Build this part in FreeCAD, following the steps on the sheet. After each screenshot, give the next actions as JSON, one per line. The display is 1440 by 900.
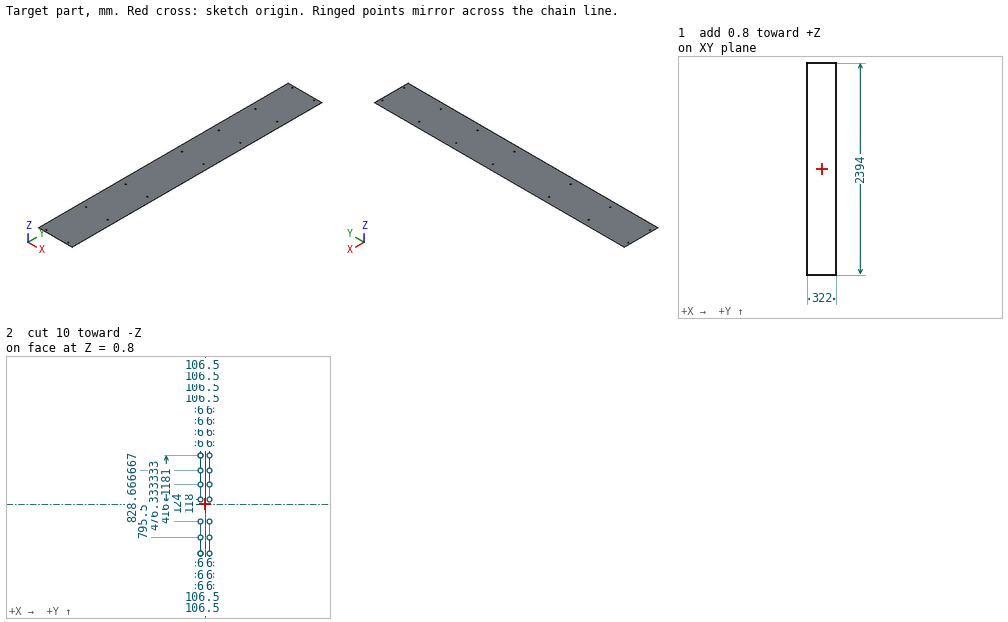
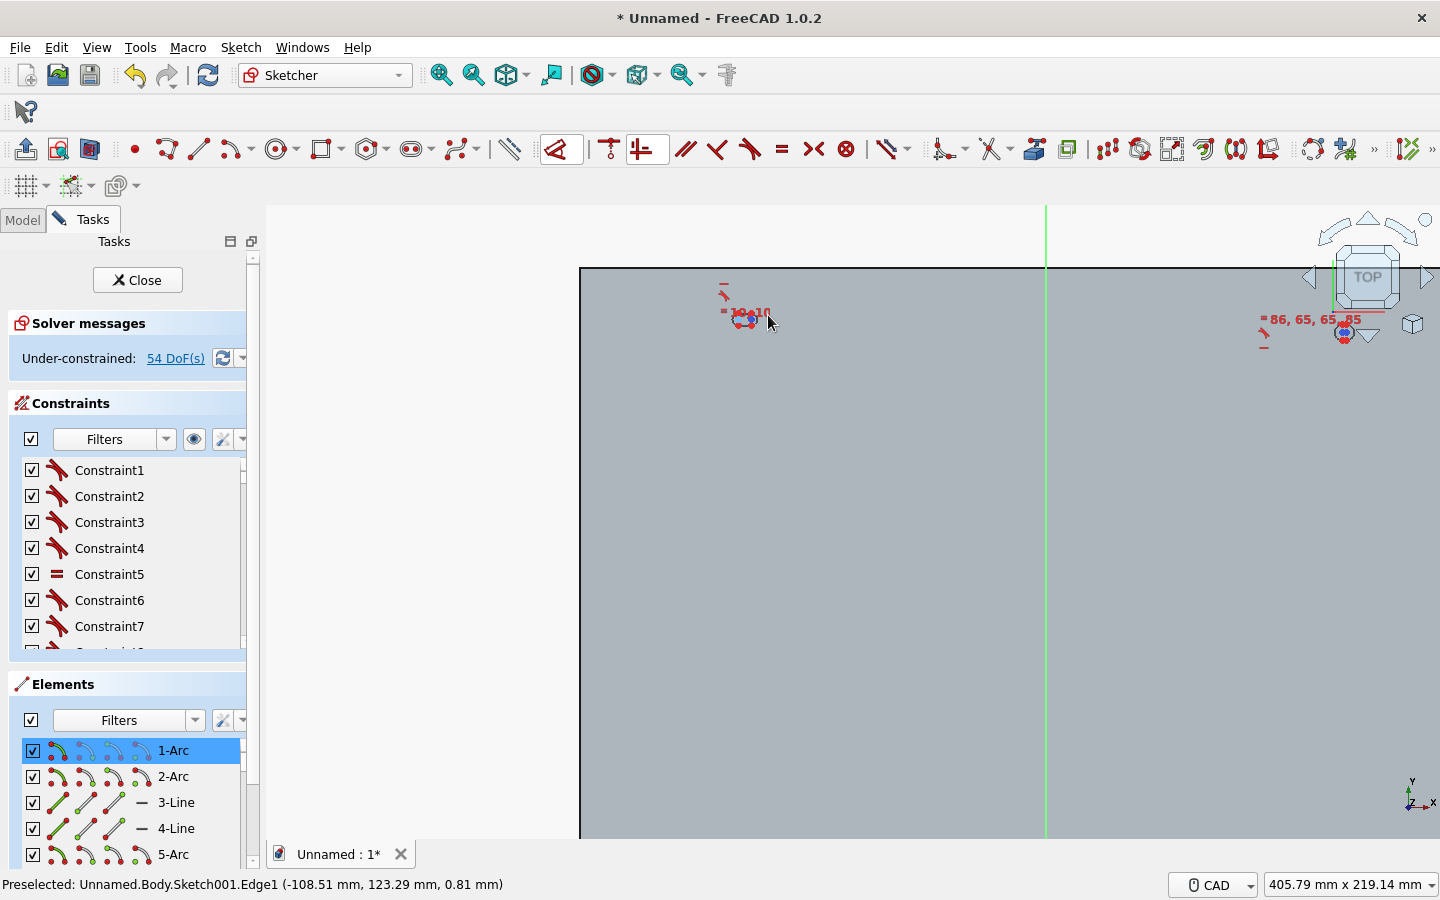
{"action": "left_click", "coordinate": [757, 320]}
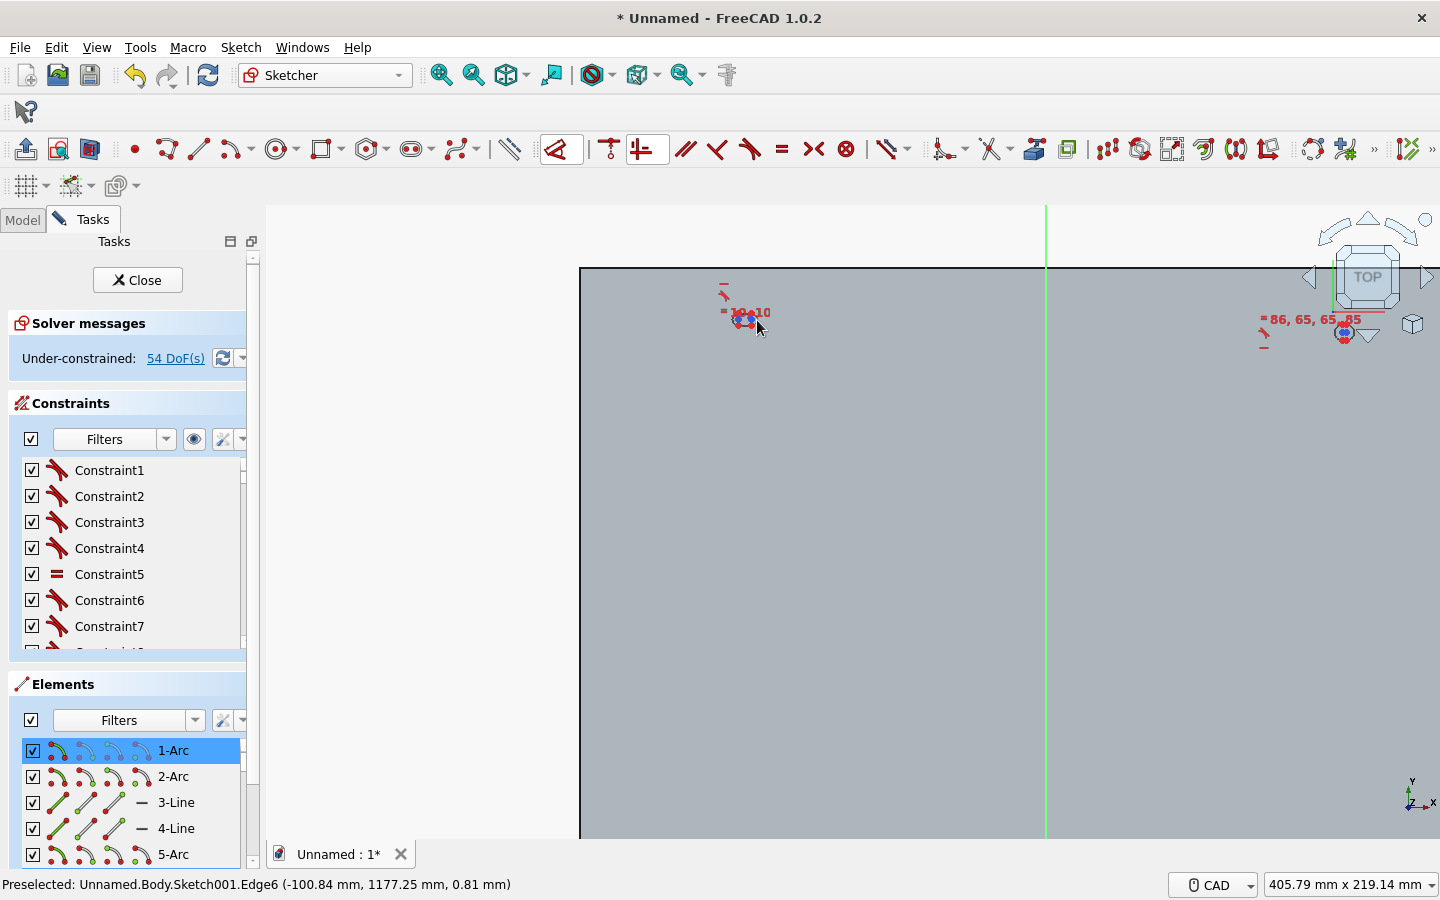
{"action": "scroll", "coordinate": [768, 314], "scroll_direction": "down", "scroll_amount": 14}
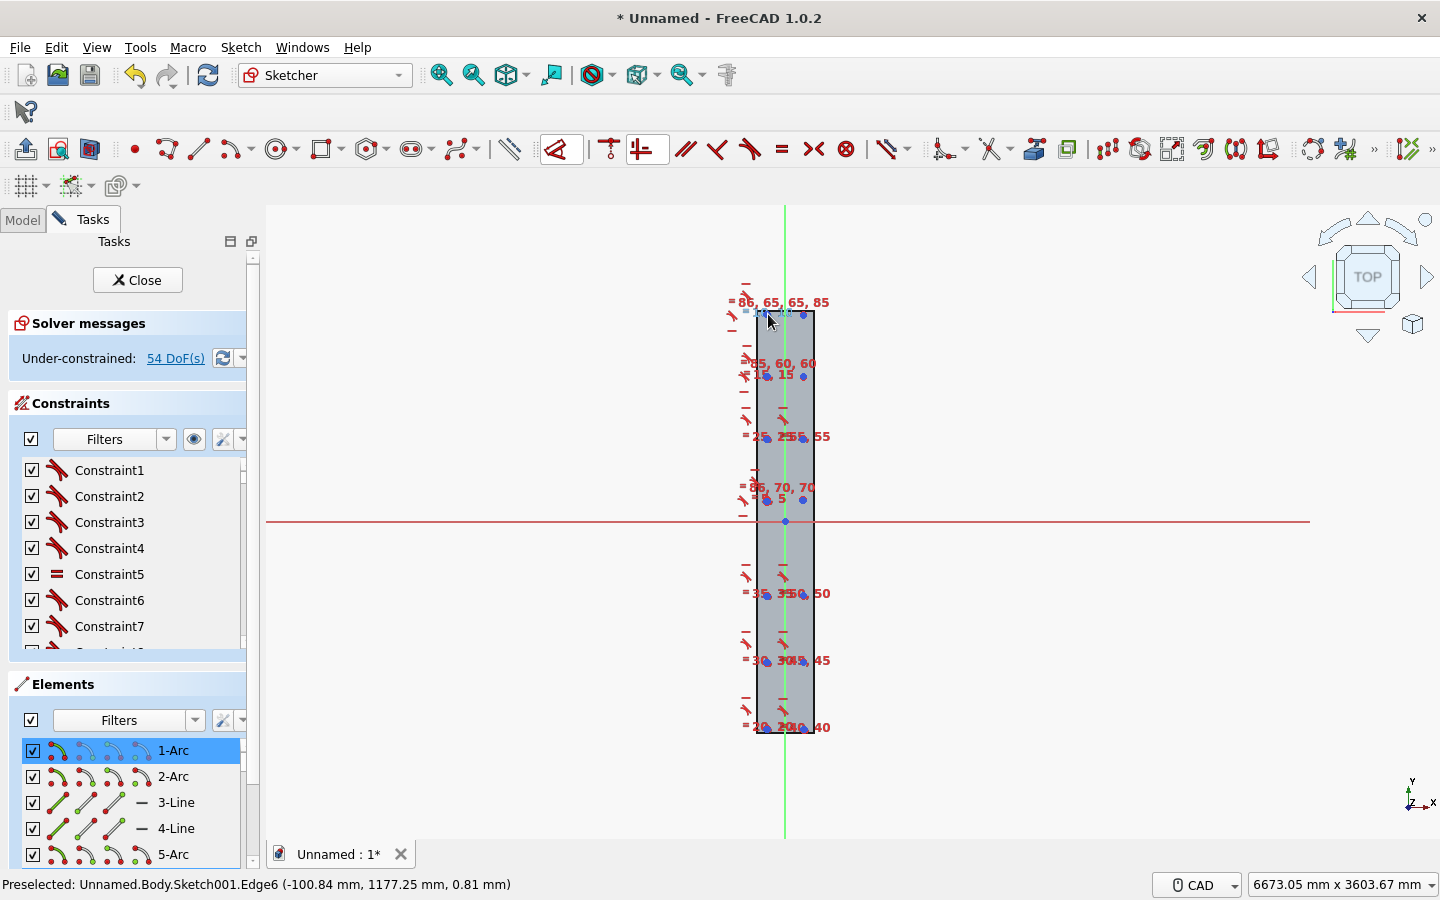
{"action": "scroll", "coordinate": [768, 377], "scroll_direction": "up", "scroll_amount": 14}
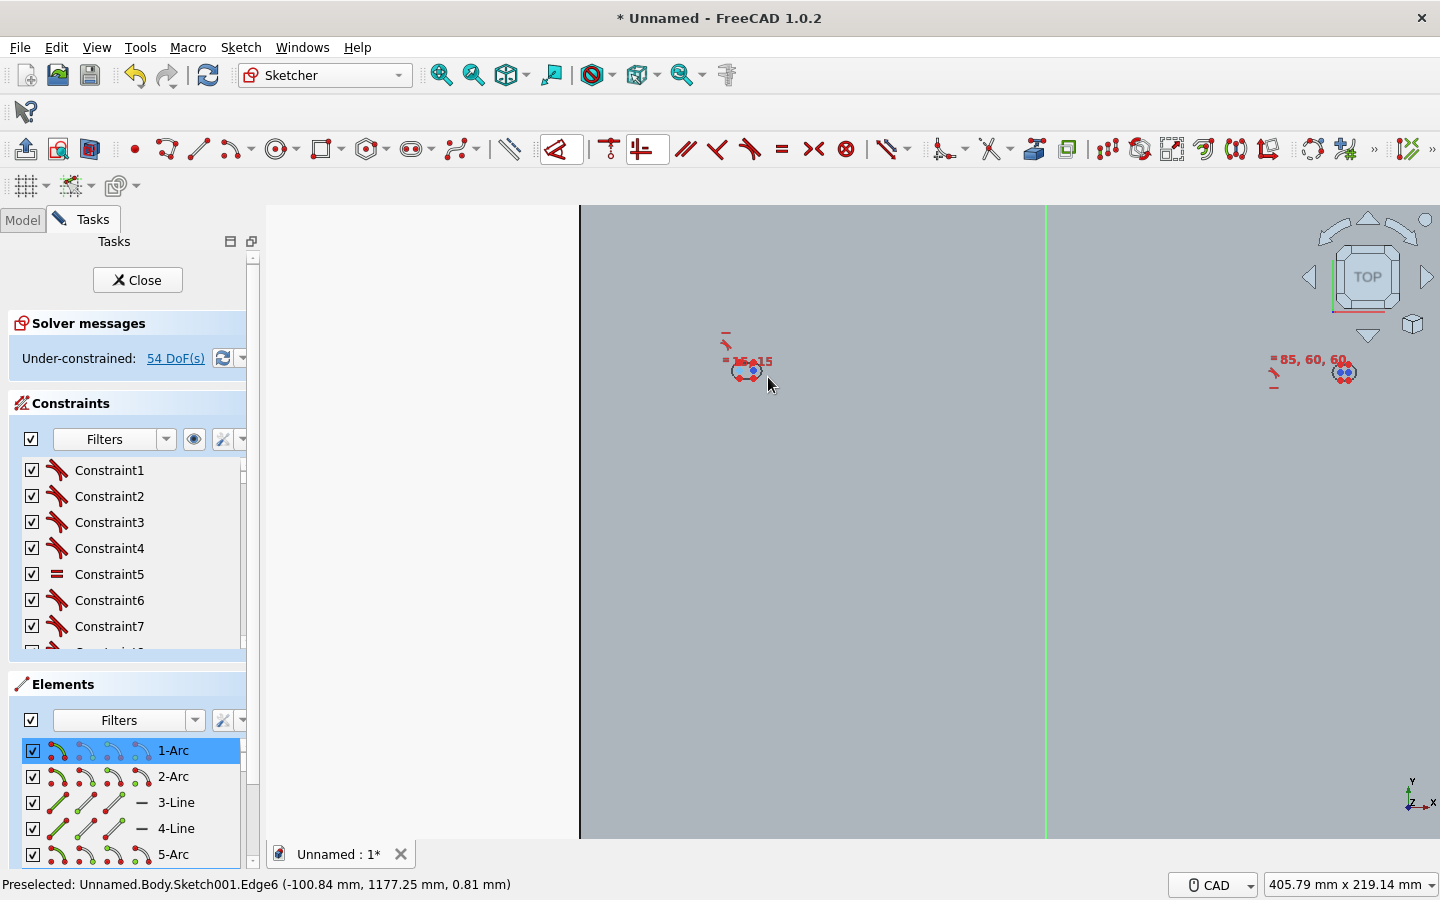
{"action": "left_click", "coordinate": [762, 371]}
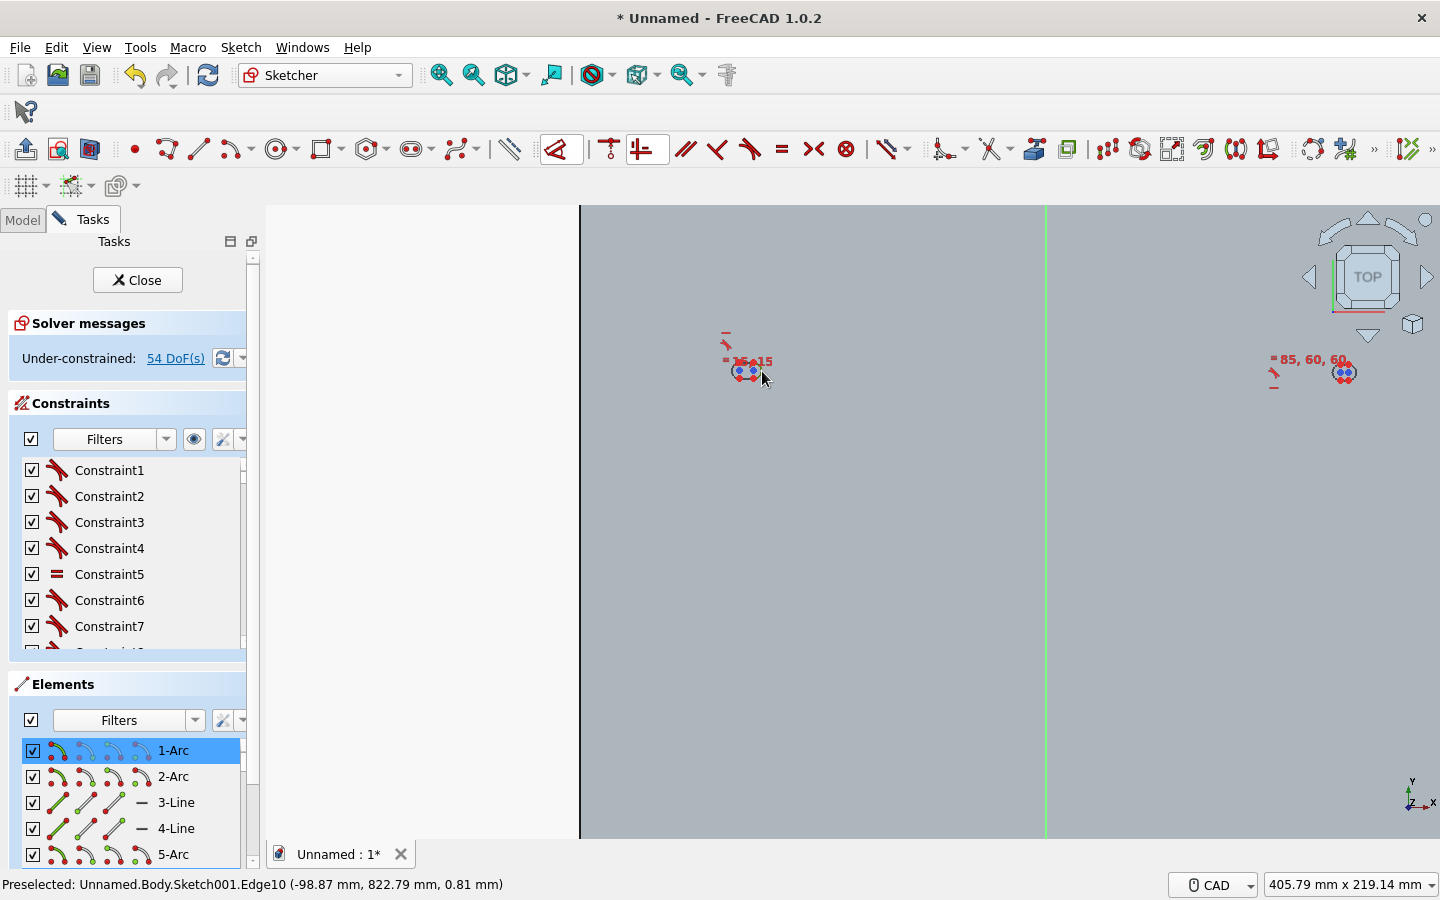
{"action": "scroll", "coordinate": [768, 377], "scroll_direction": "down", "scroll_amount": 14}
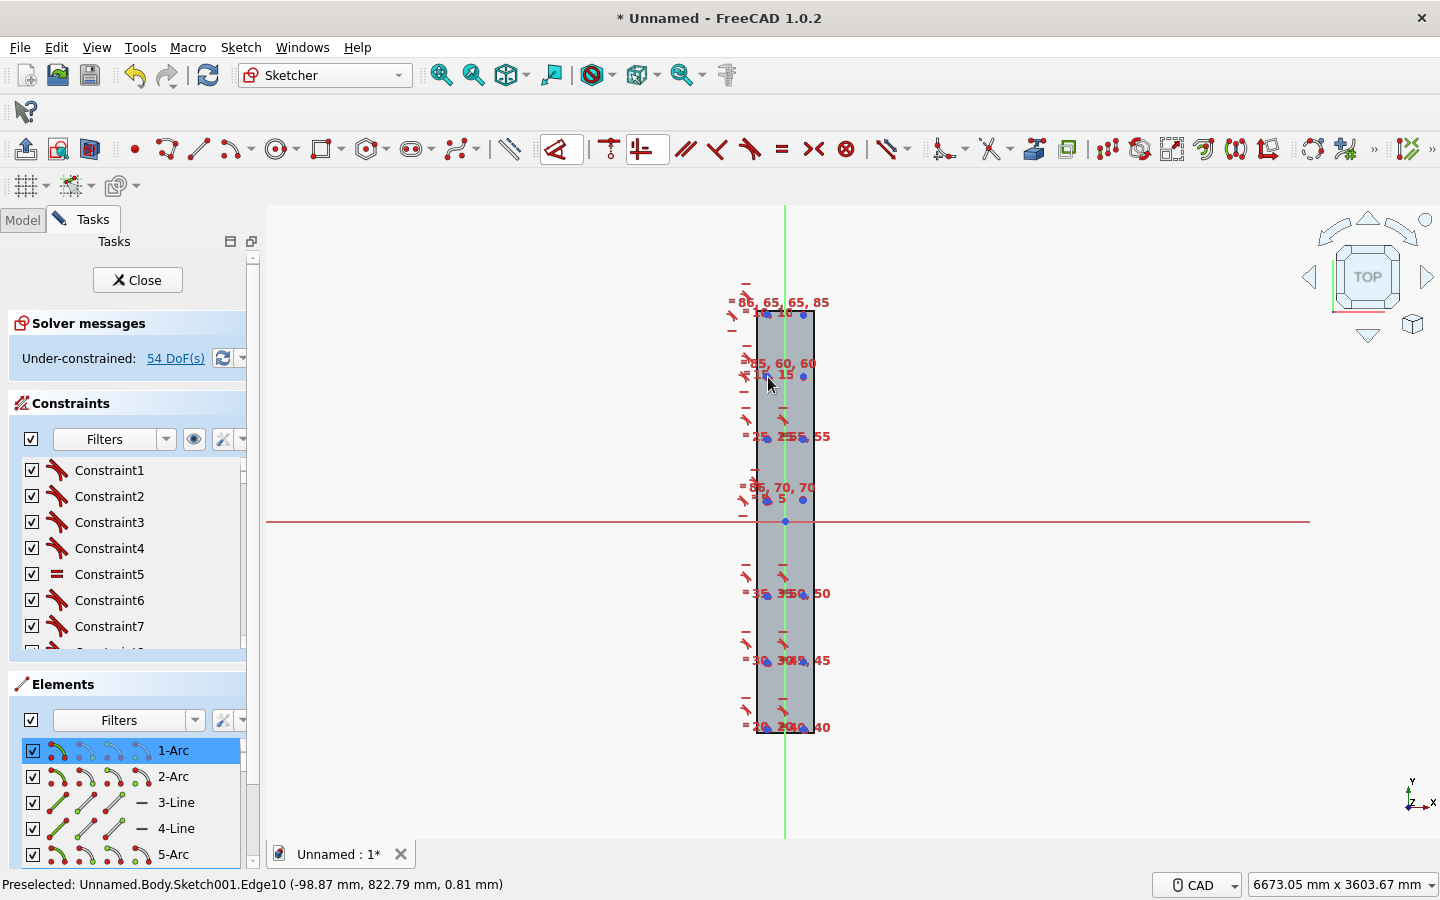
{"action": "scroll", "coordinate": [768, 729], "scroll_direction": "up", "scroll_amount": 14}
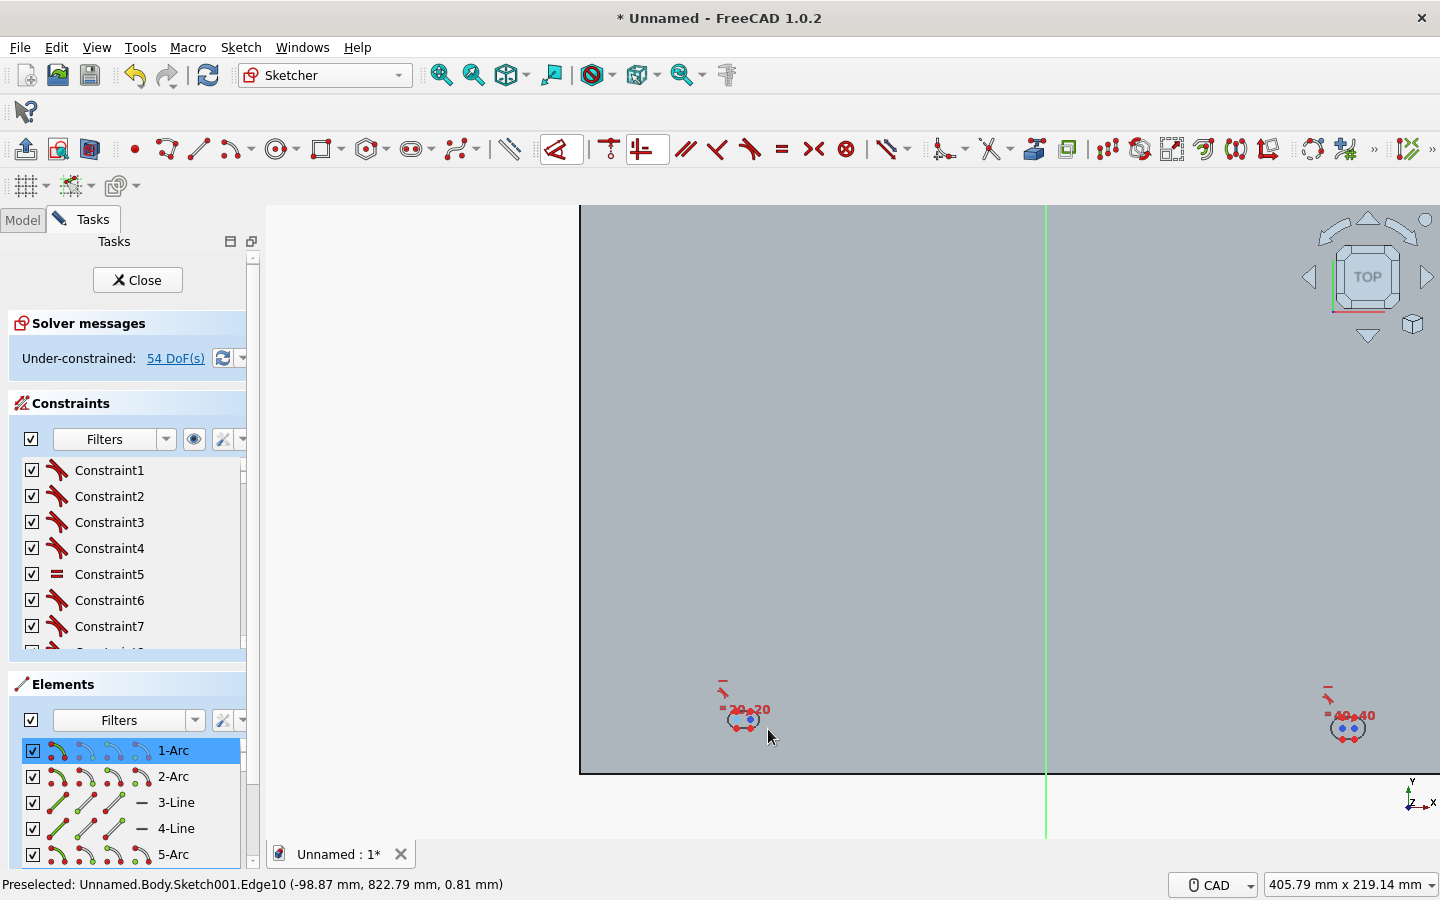
{"action": "left_click", "coordinate": [759, 720]}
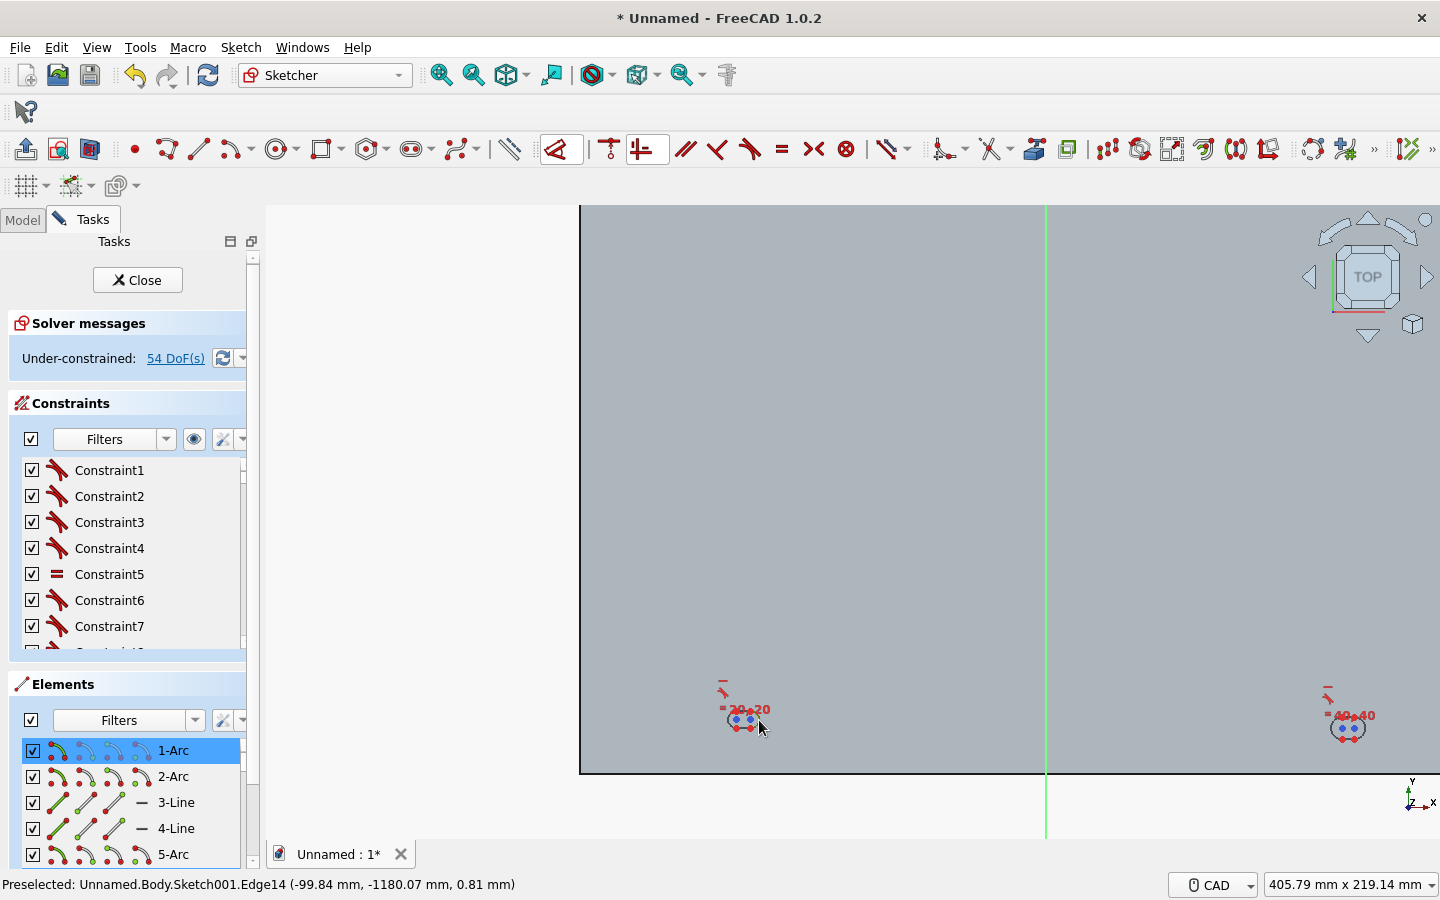
{"action": "scroll", "coordinate": [768, 730], "scroll_direction": "down", "scroll_amount": 14}